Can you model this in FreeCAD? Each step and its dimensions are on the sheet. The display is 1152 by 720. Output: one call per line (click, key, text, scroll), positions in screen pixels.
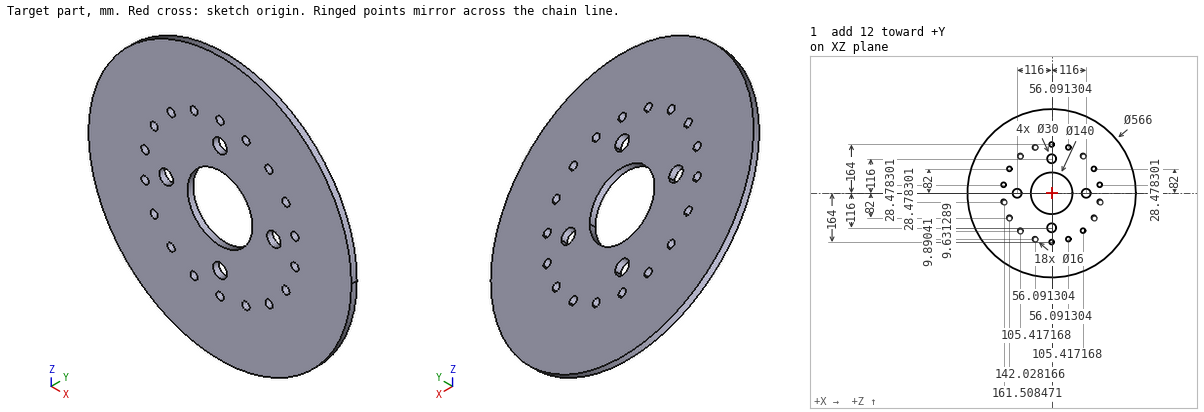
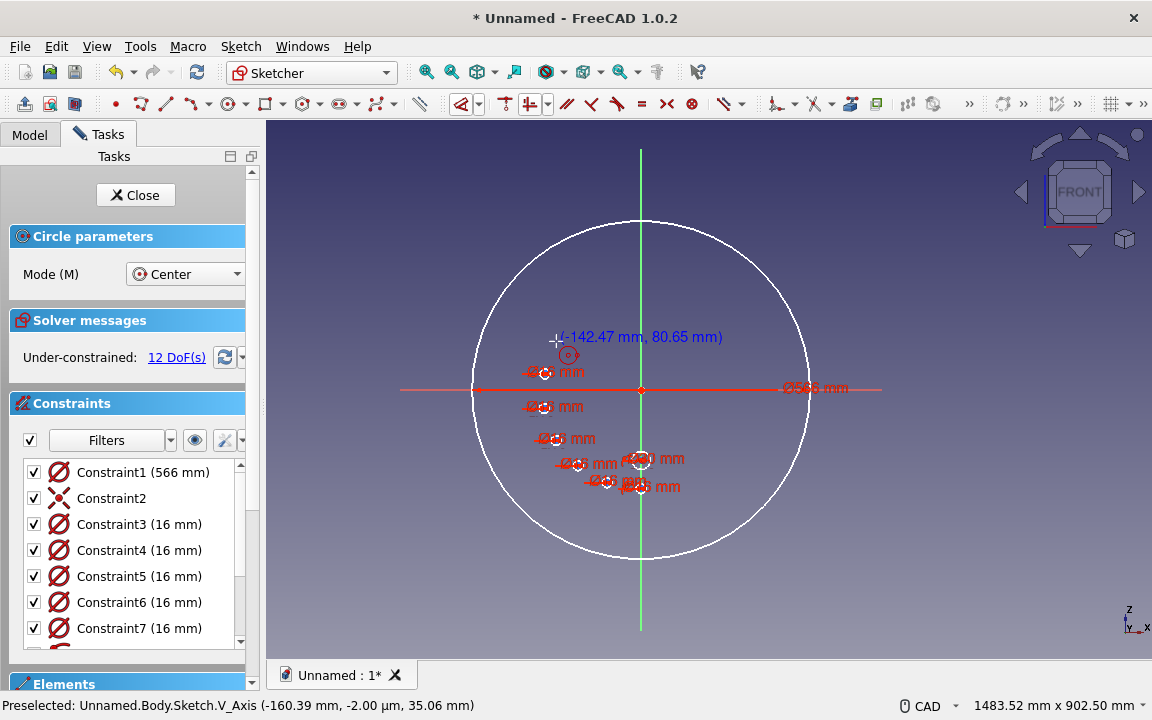
click(556, 341)
move(560, 338)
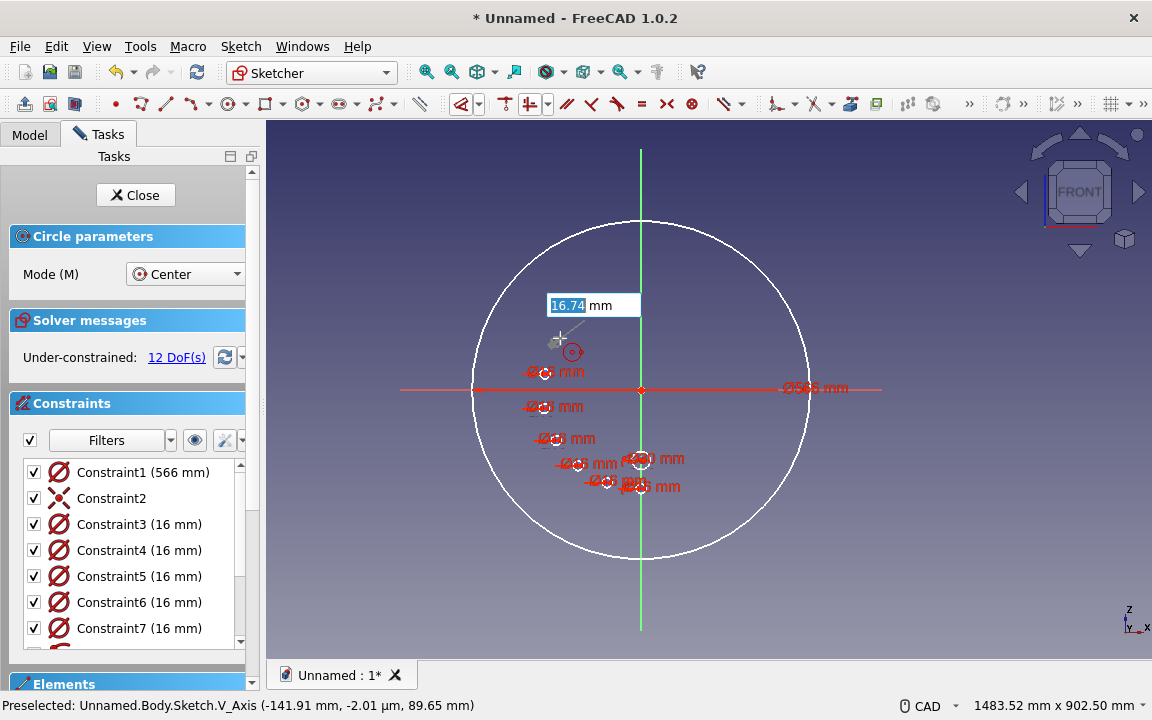
text(16)
key(Return)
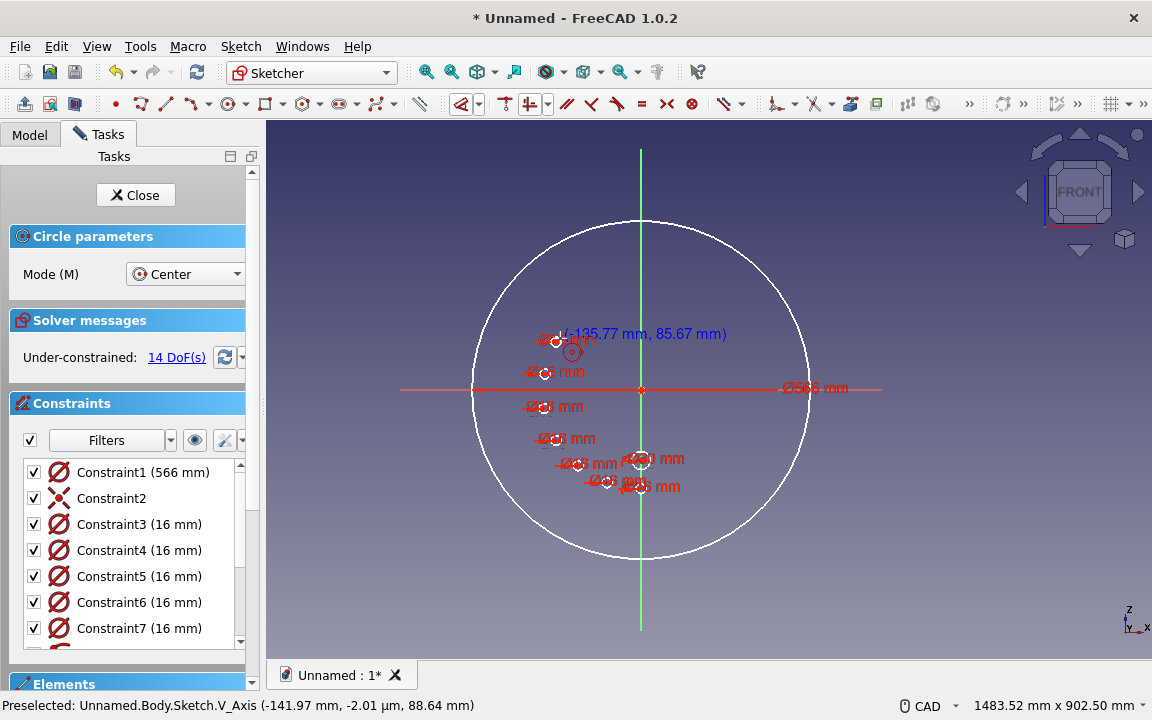
scroll(572, 390, up, 5)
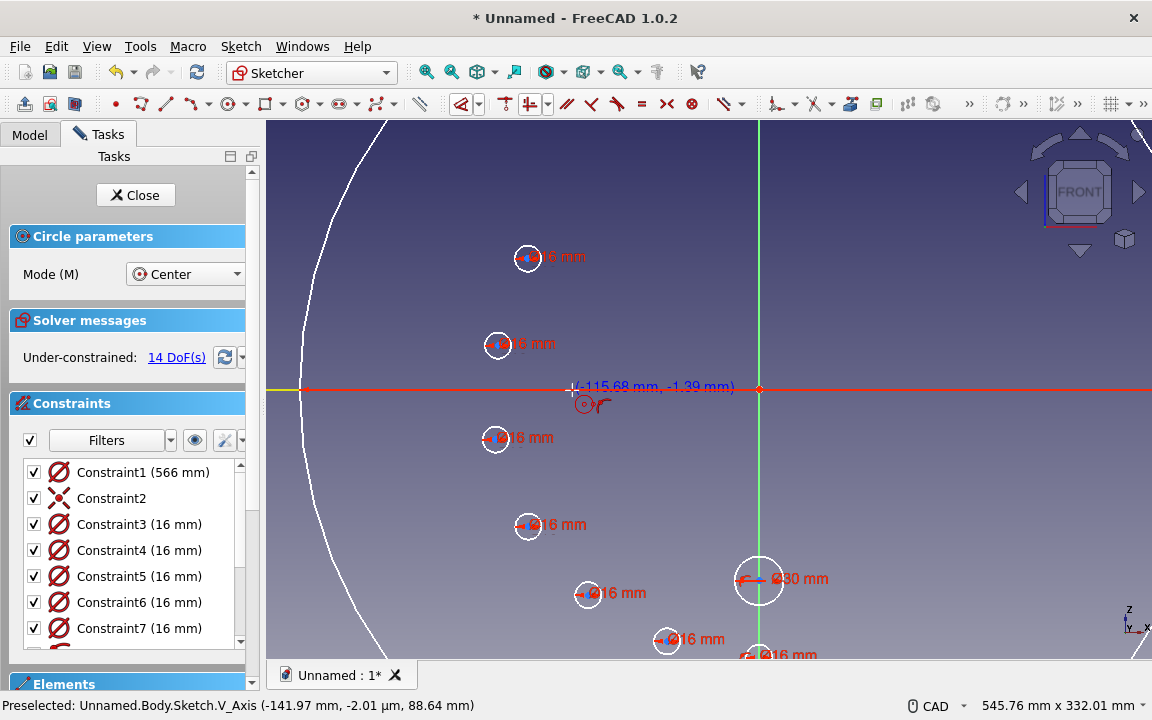
click(571, 390)
move(588, 372)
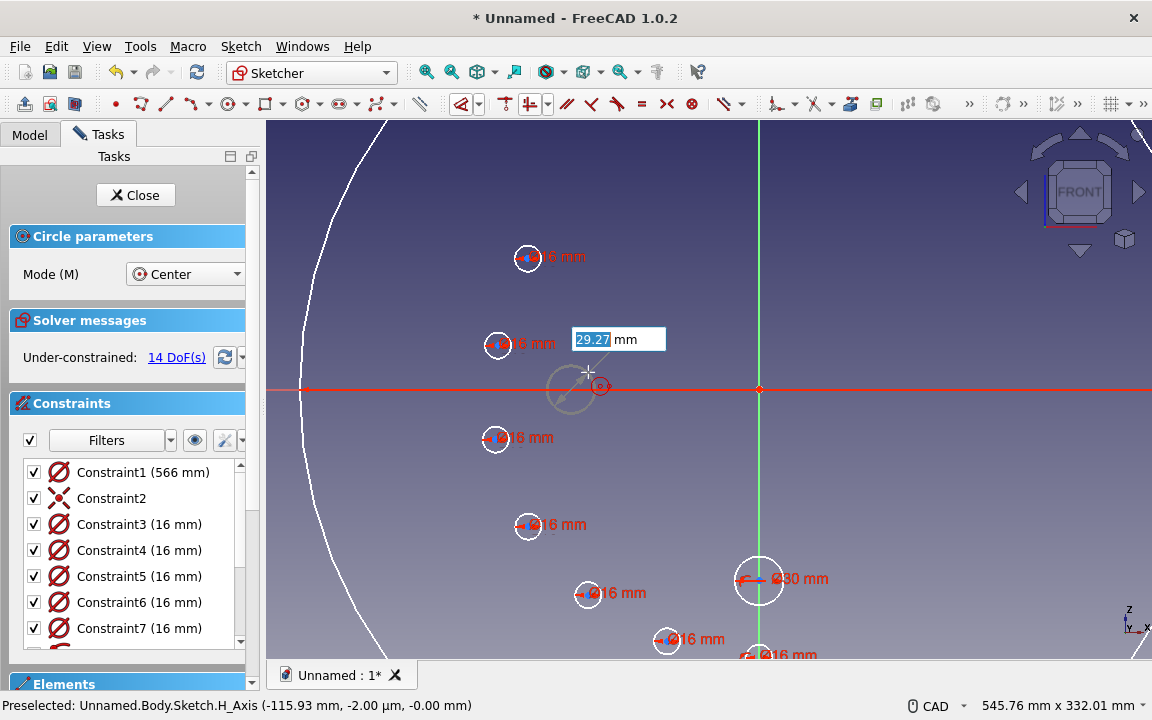
text(30)
key(Return)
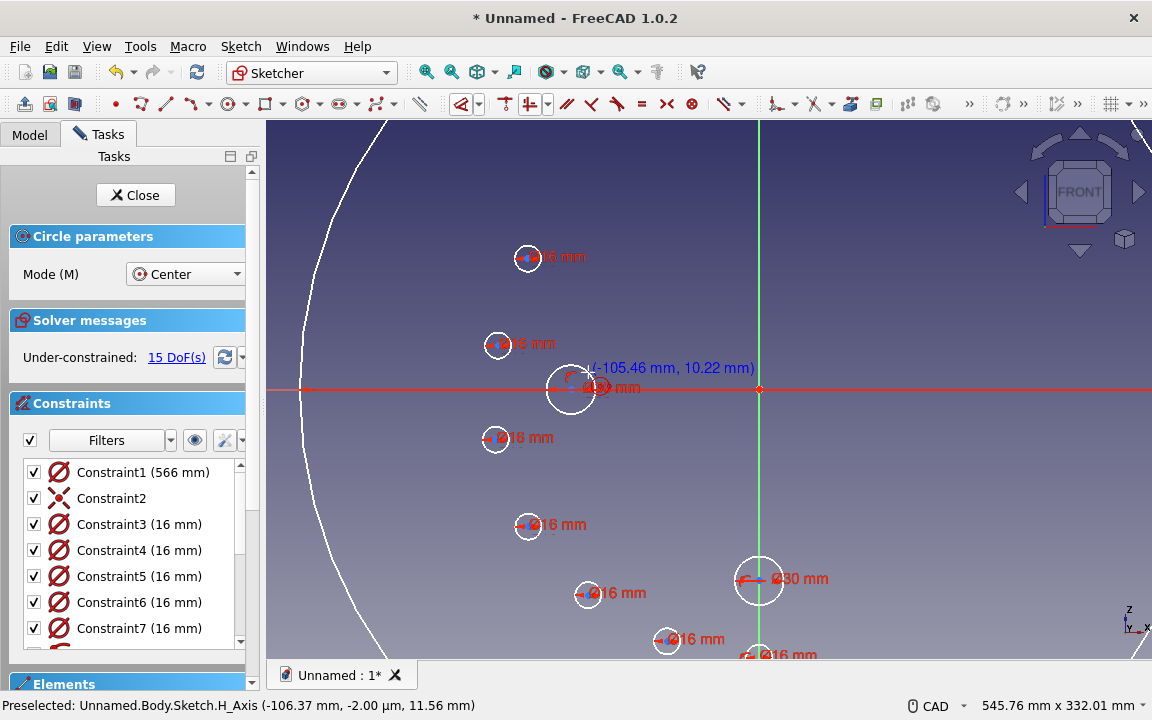
scroll(588, 186, up, 3)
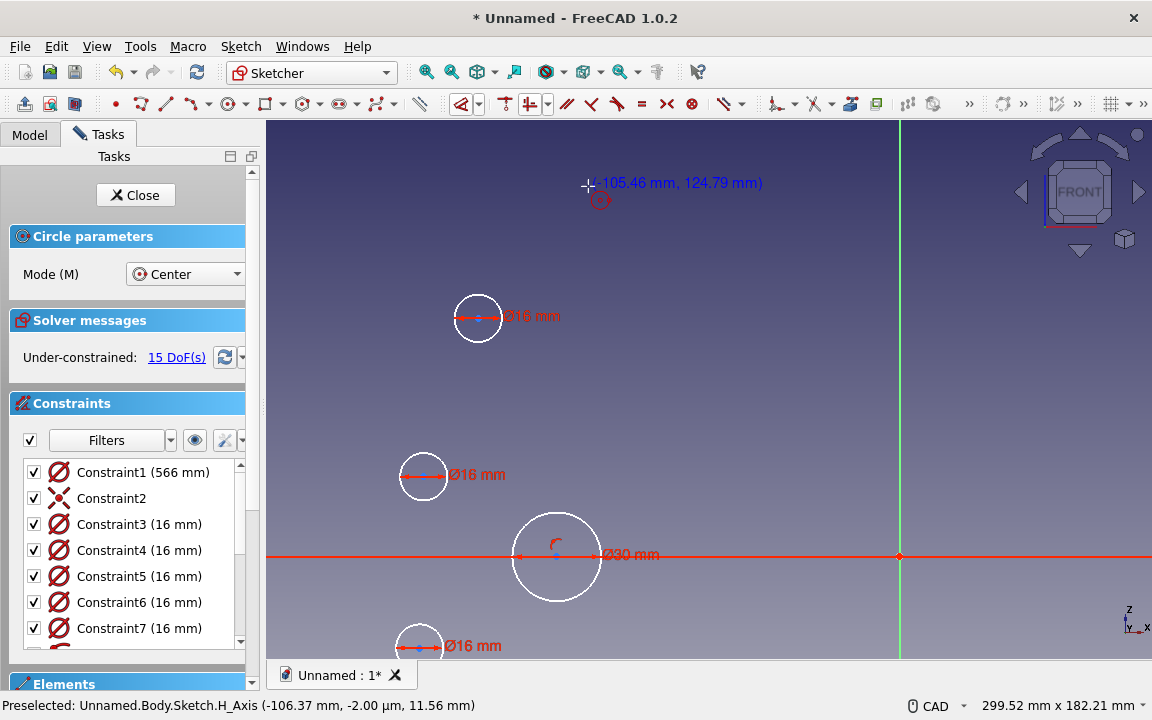
scroll(575, 347, down, 8)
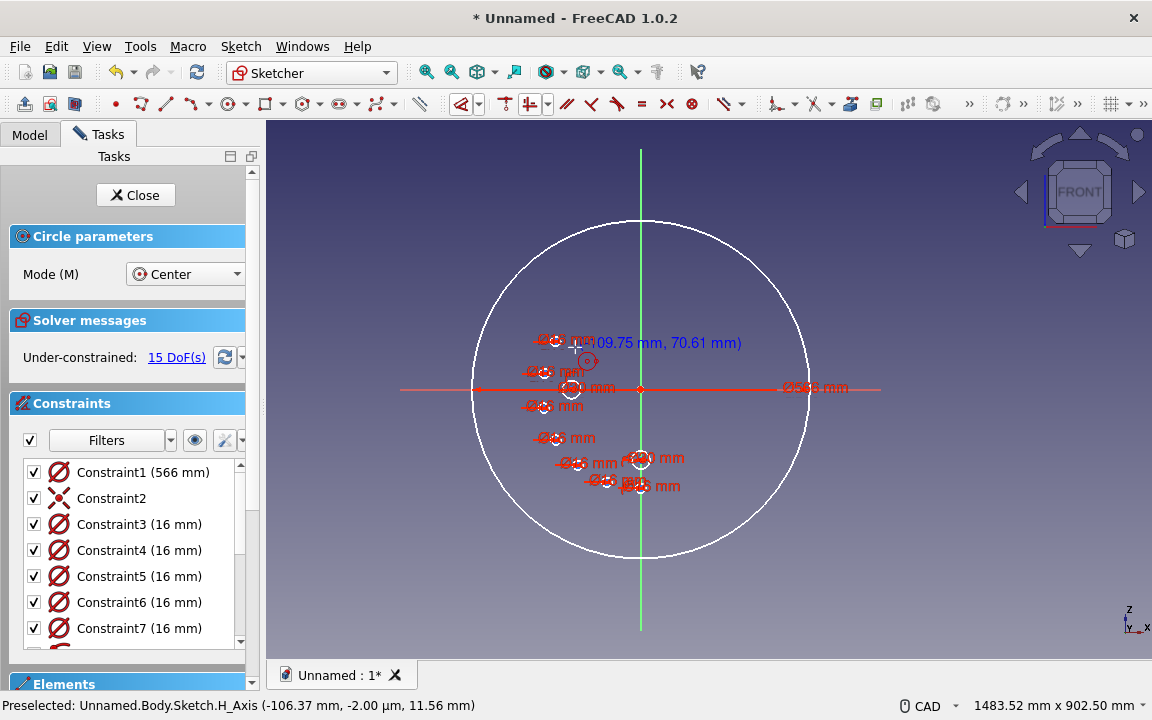
click(578, 315)
move(581, 311)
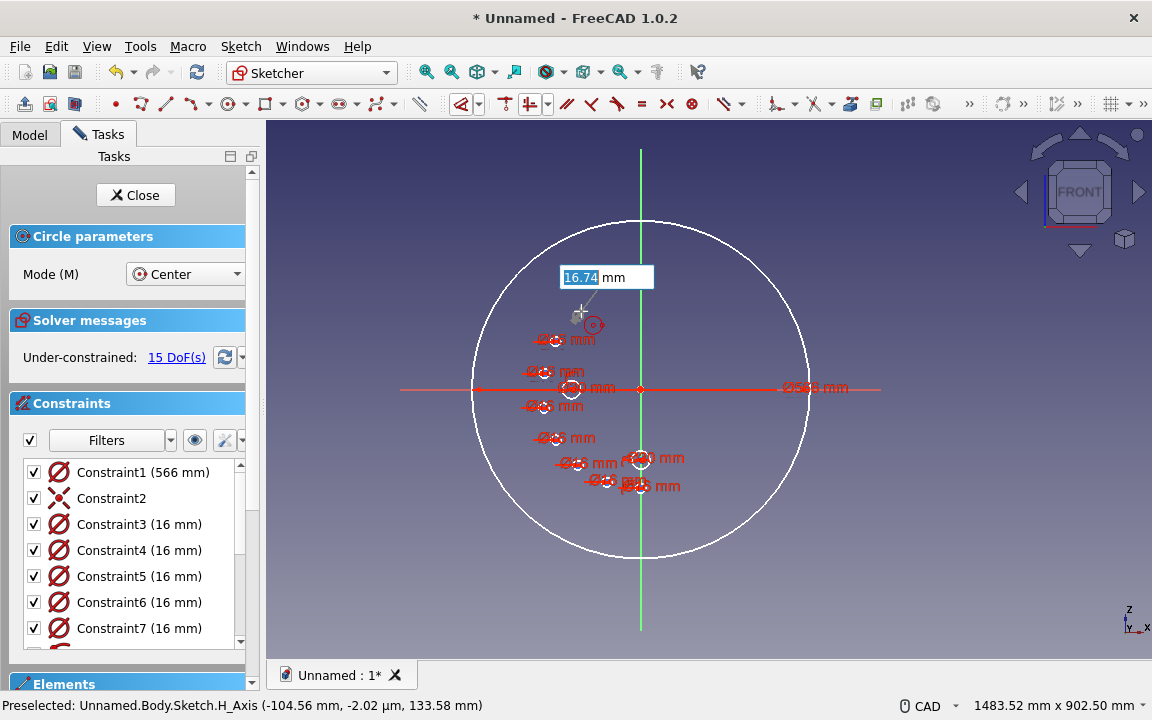
text(16)
key(Return)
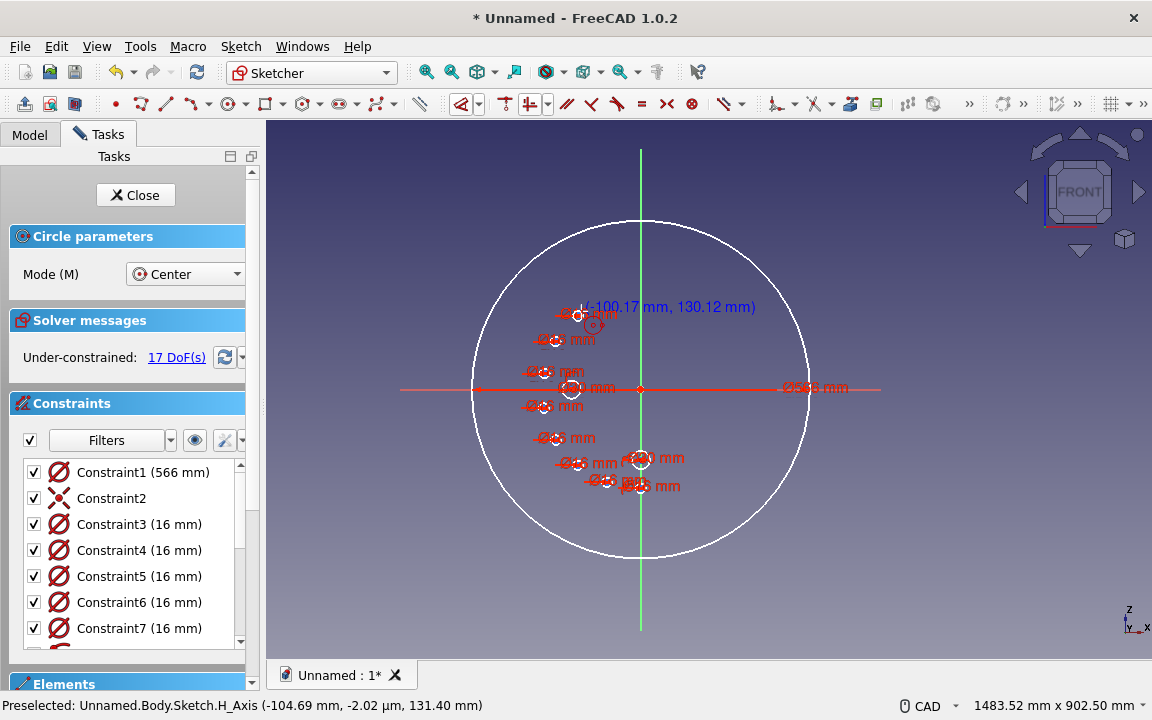
scroll(607, 298, up, 8)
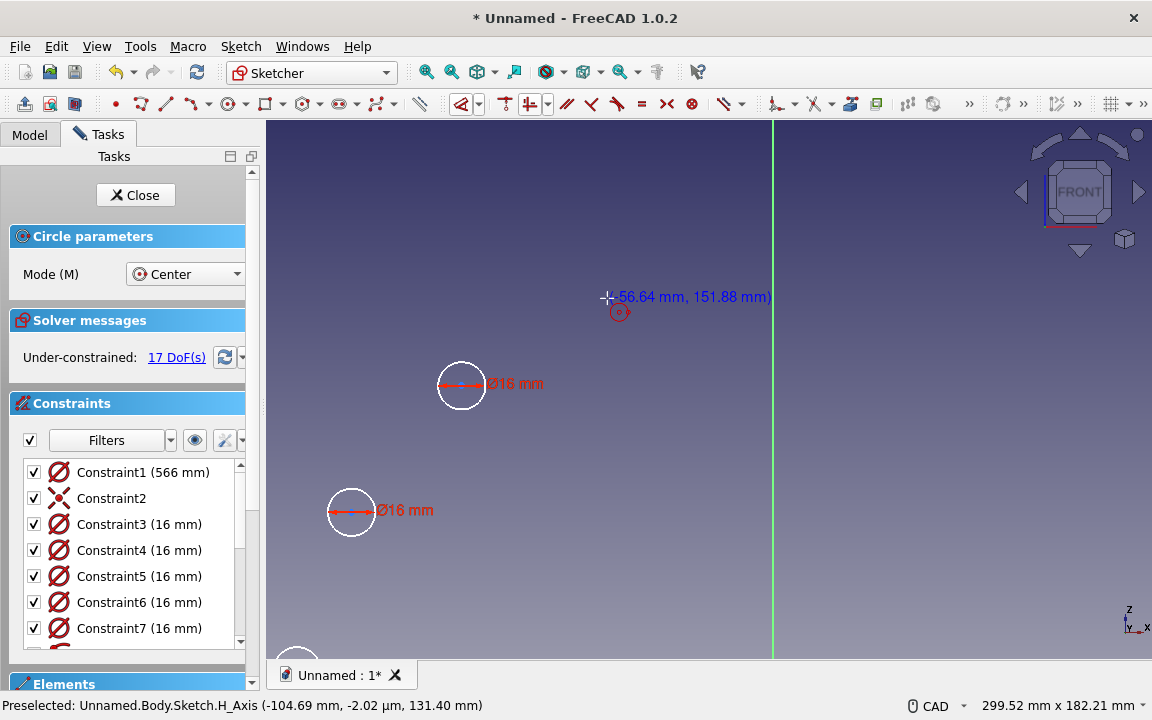
scroll(607, 298, down, 8)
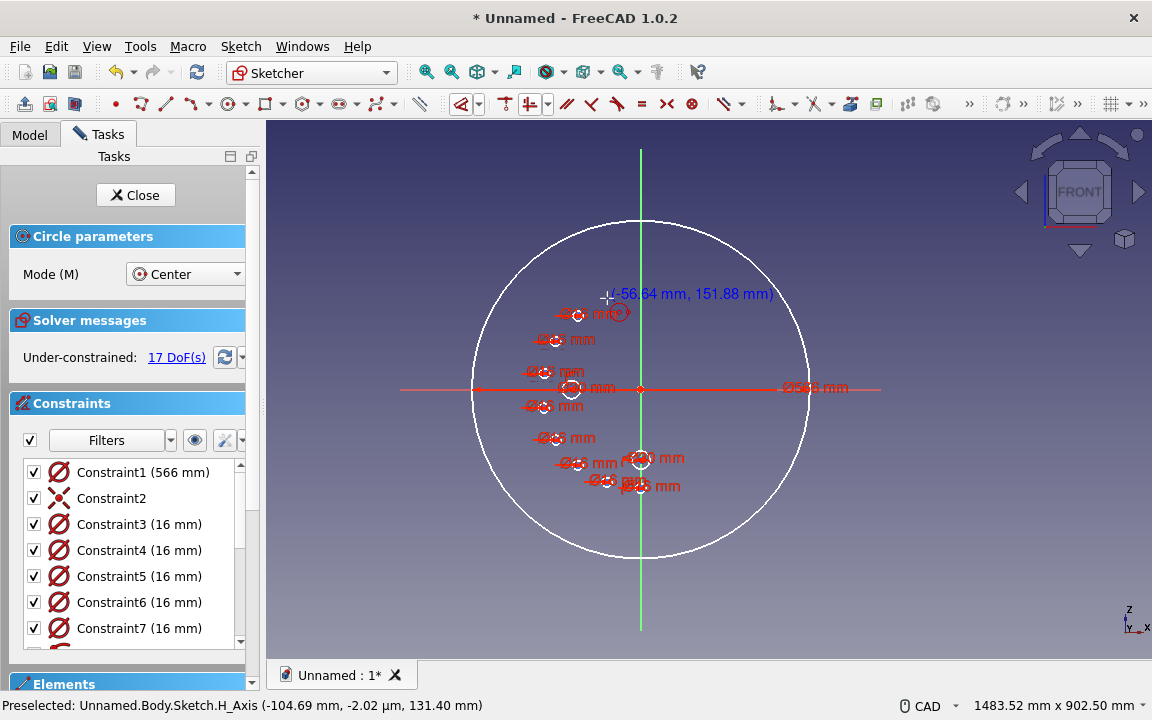
click(607, 298)
move(611, 294)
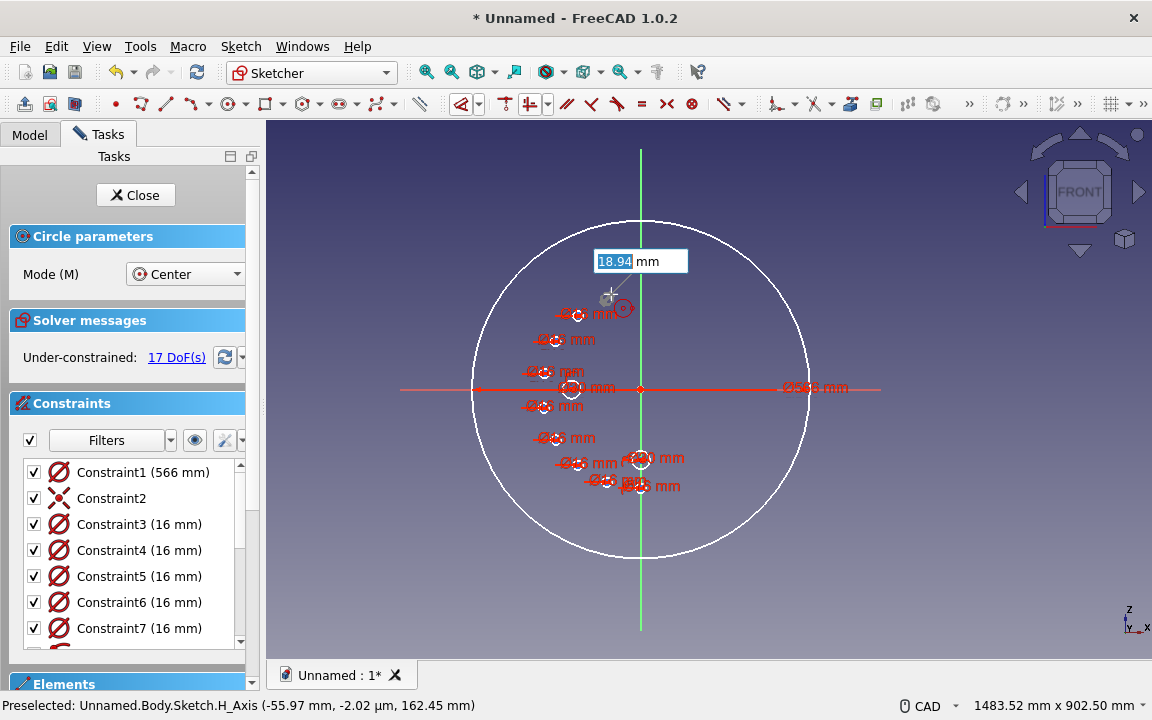
text(16)
key(Return)